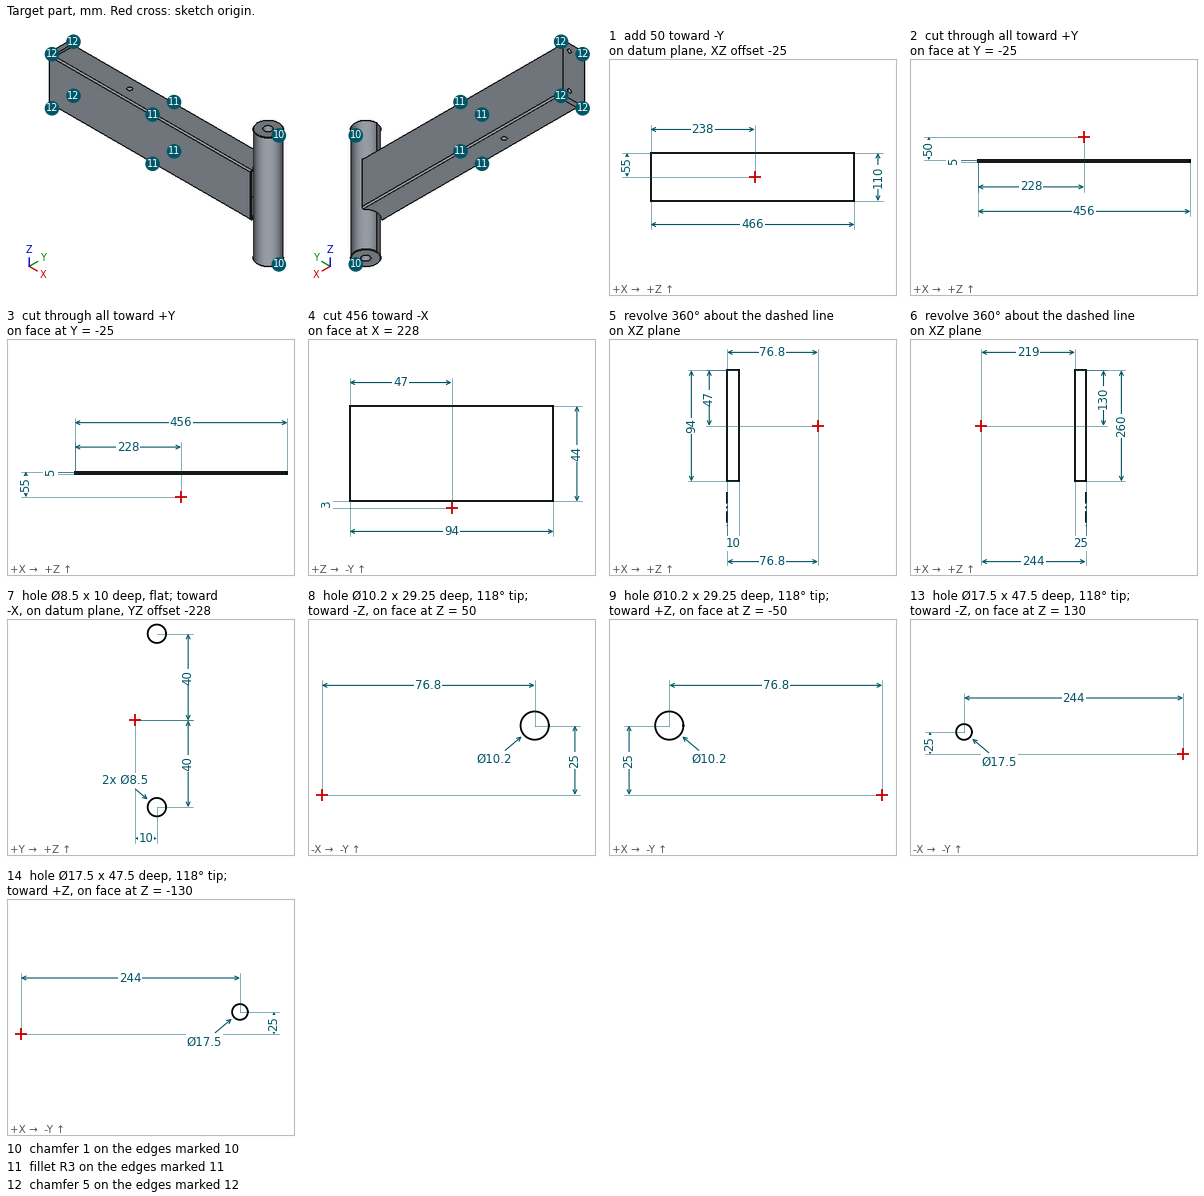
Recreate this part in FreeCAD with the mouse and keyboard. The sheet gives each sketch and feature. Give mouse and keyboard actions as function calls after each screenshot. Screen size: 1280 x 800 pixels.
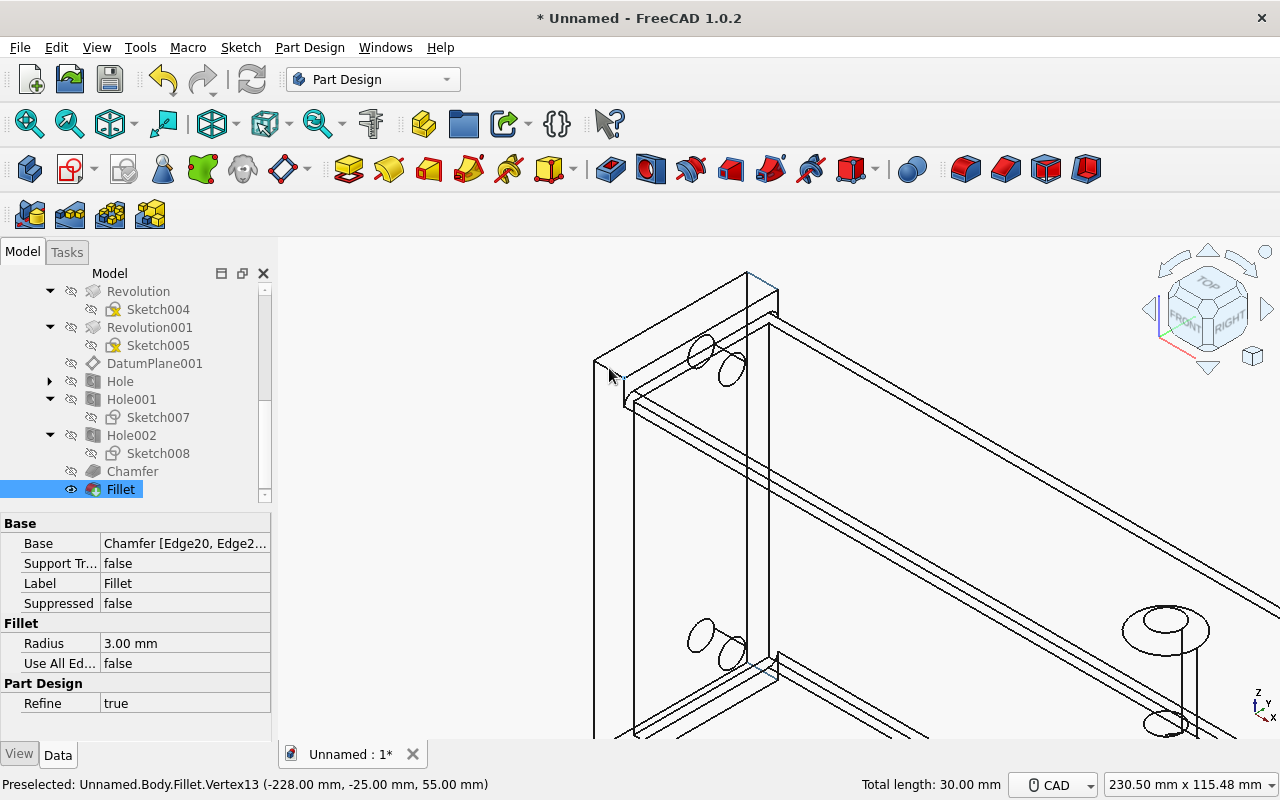
click(609, 368, ctrl)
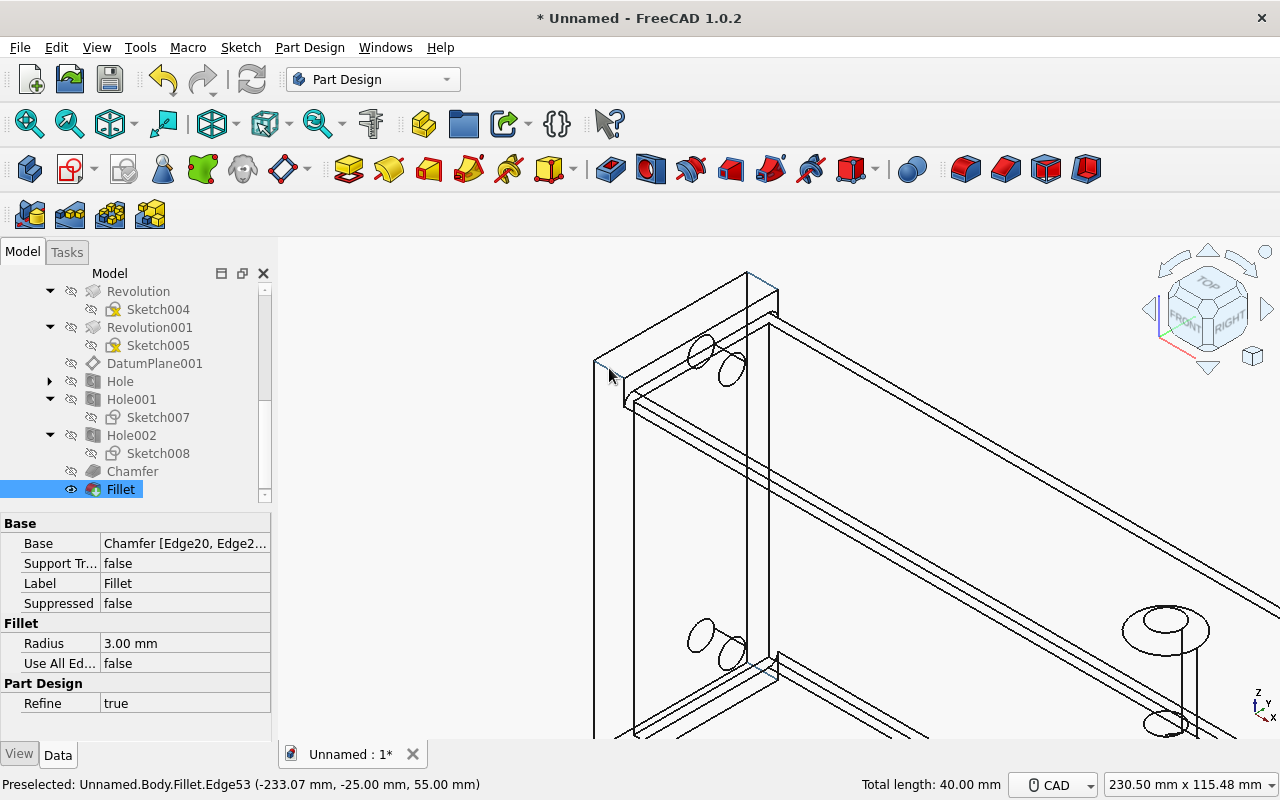
key(v)
key(1)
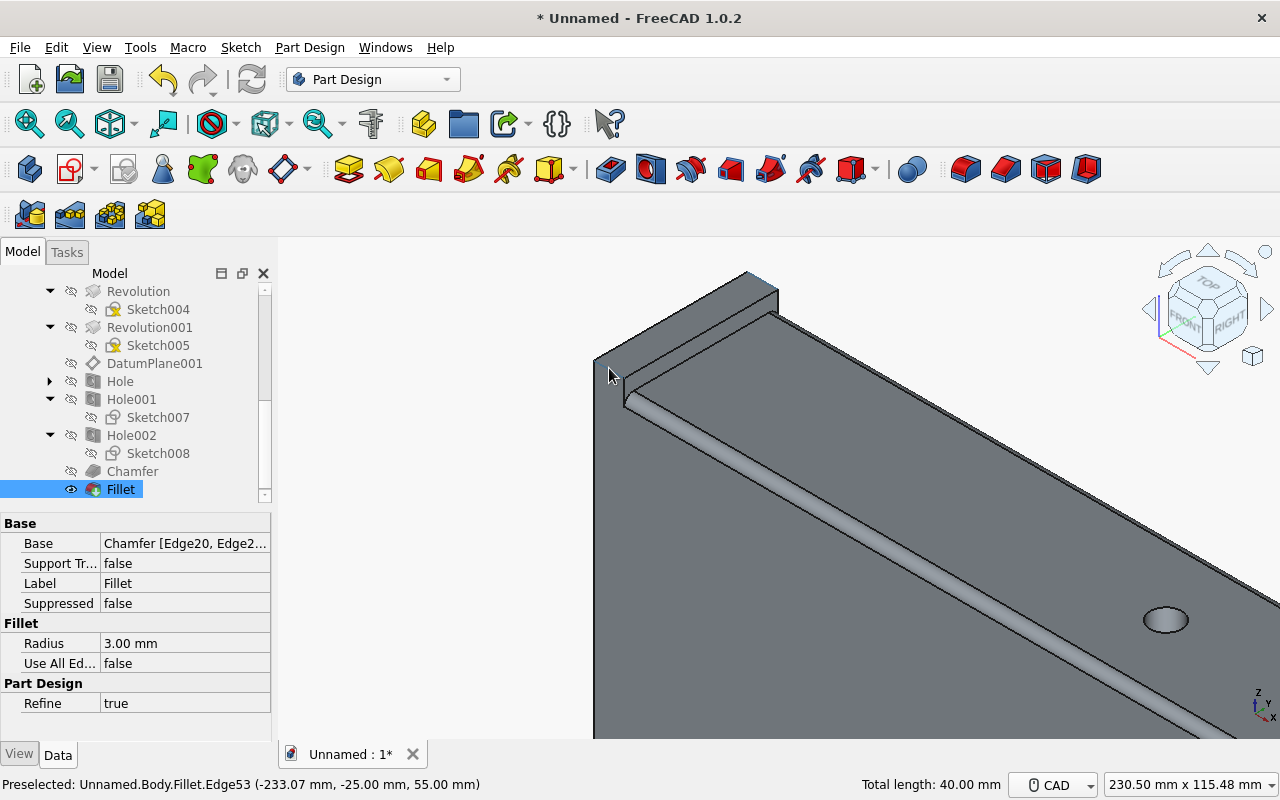
click(1006, 170)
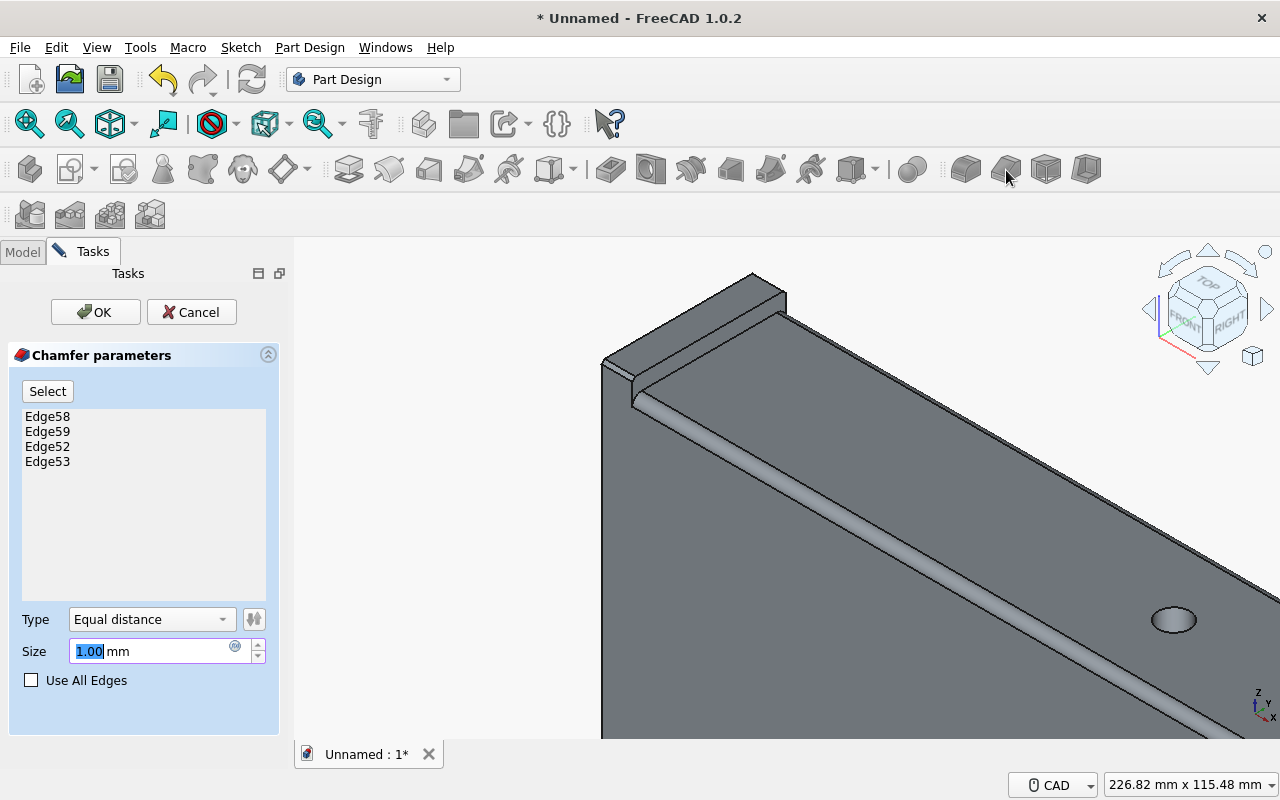
text(5)
key(Tab)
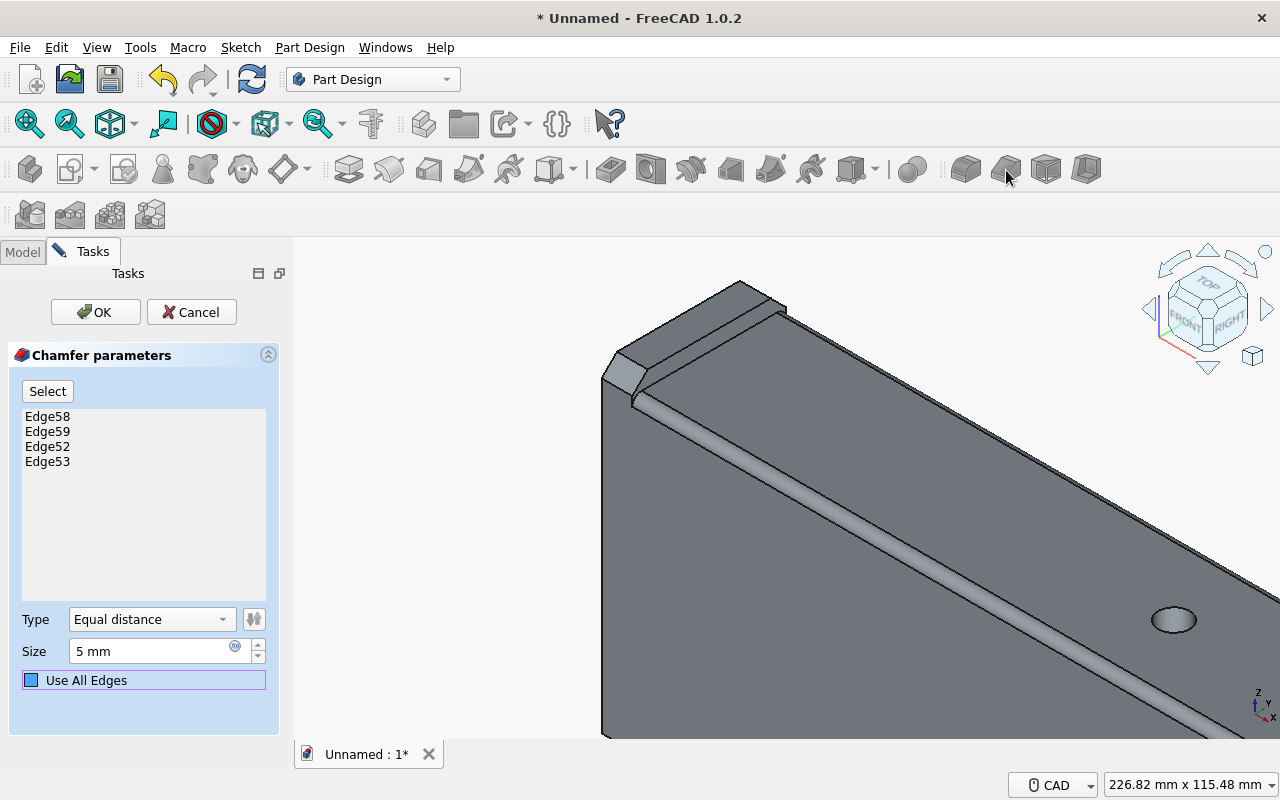
click(96, 312)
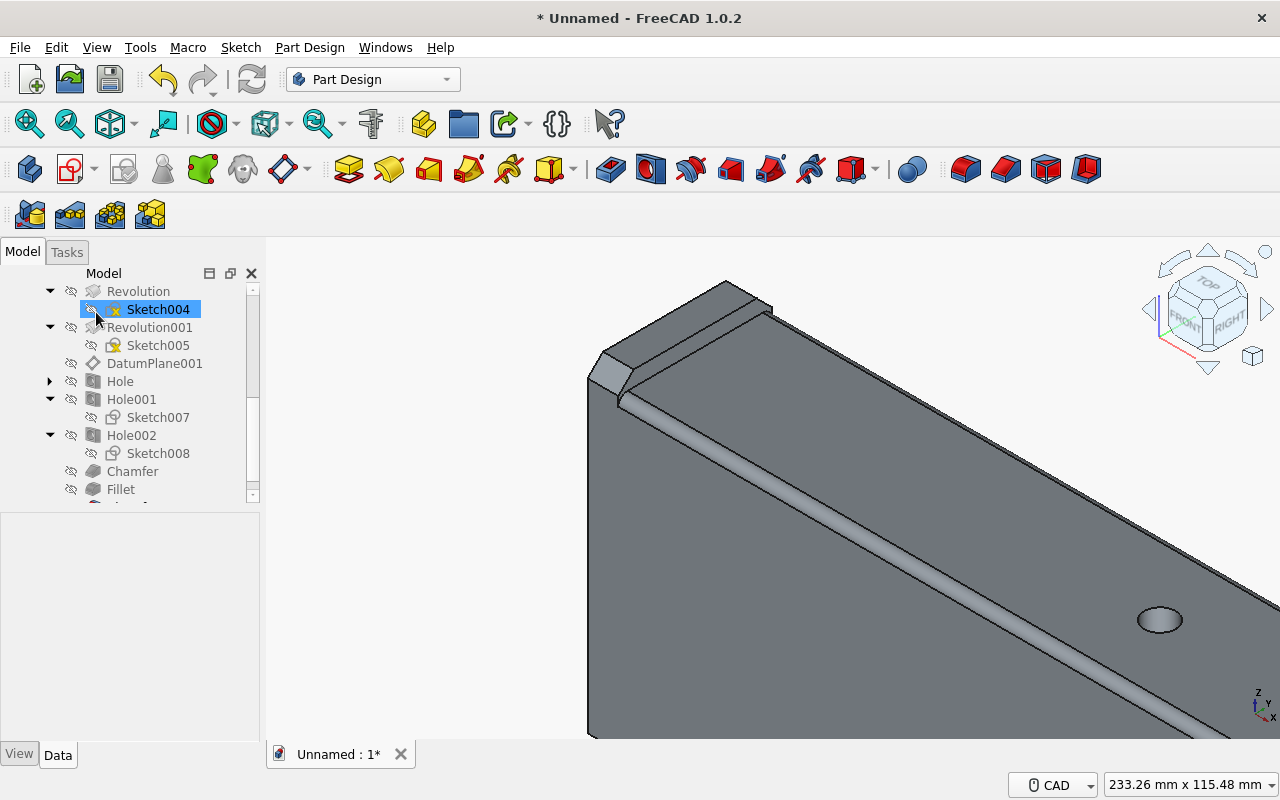
click(30, 124)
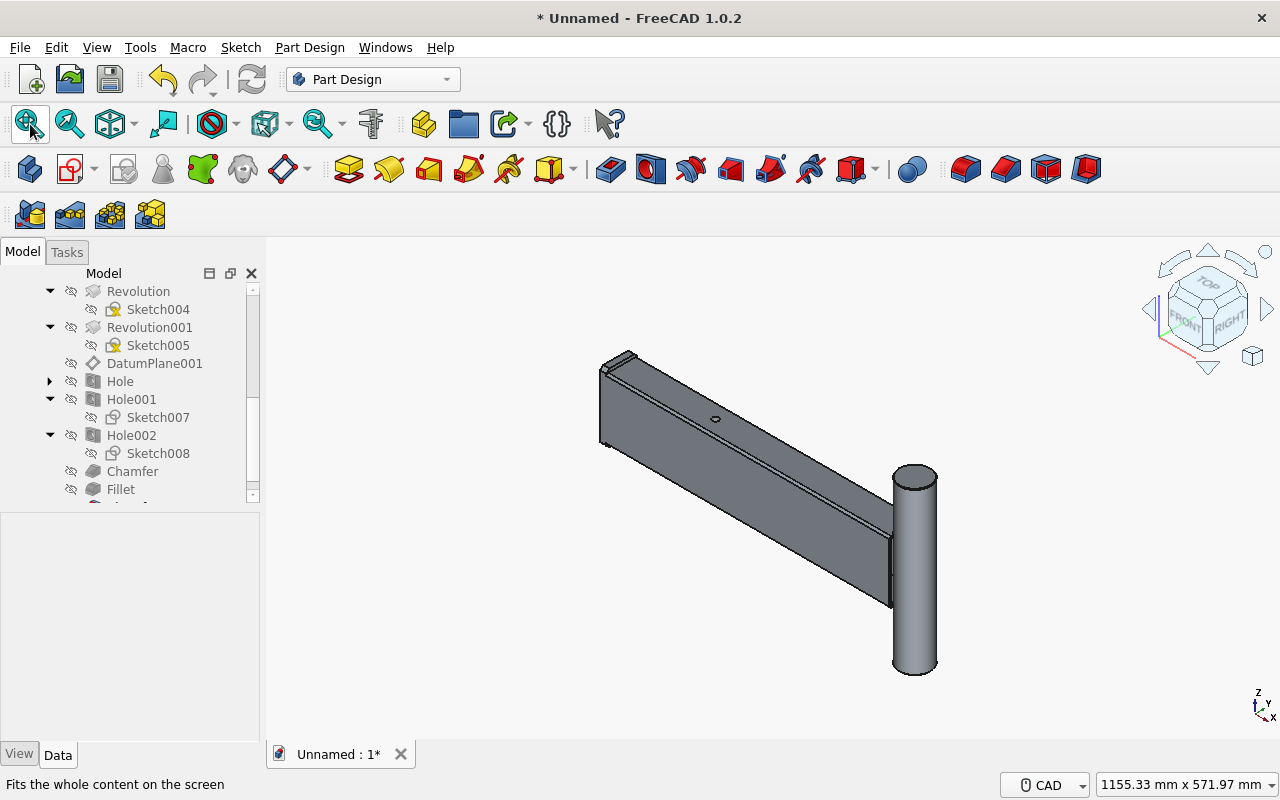
click(915, 476)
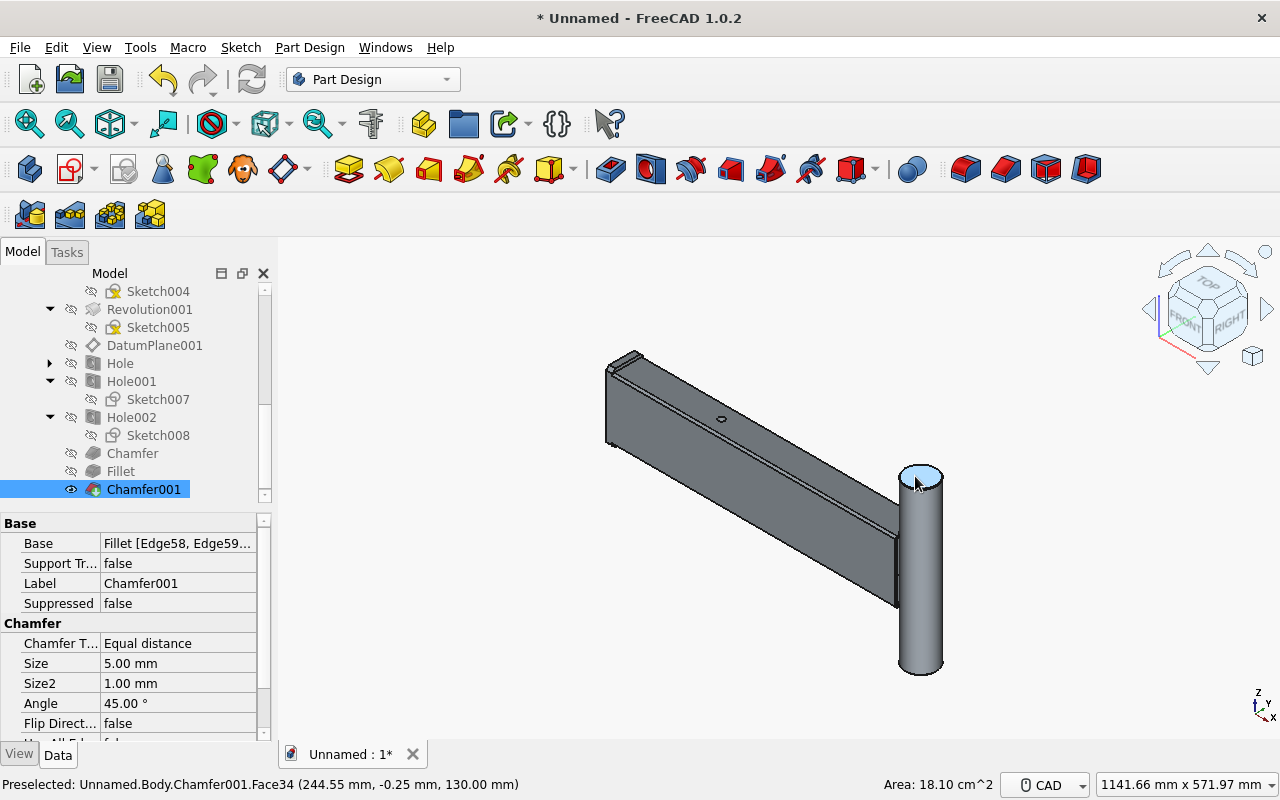
click(70, 170)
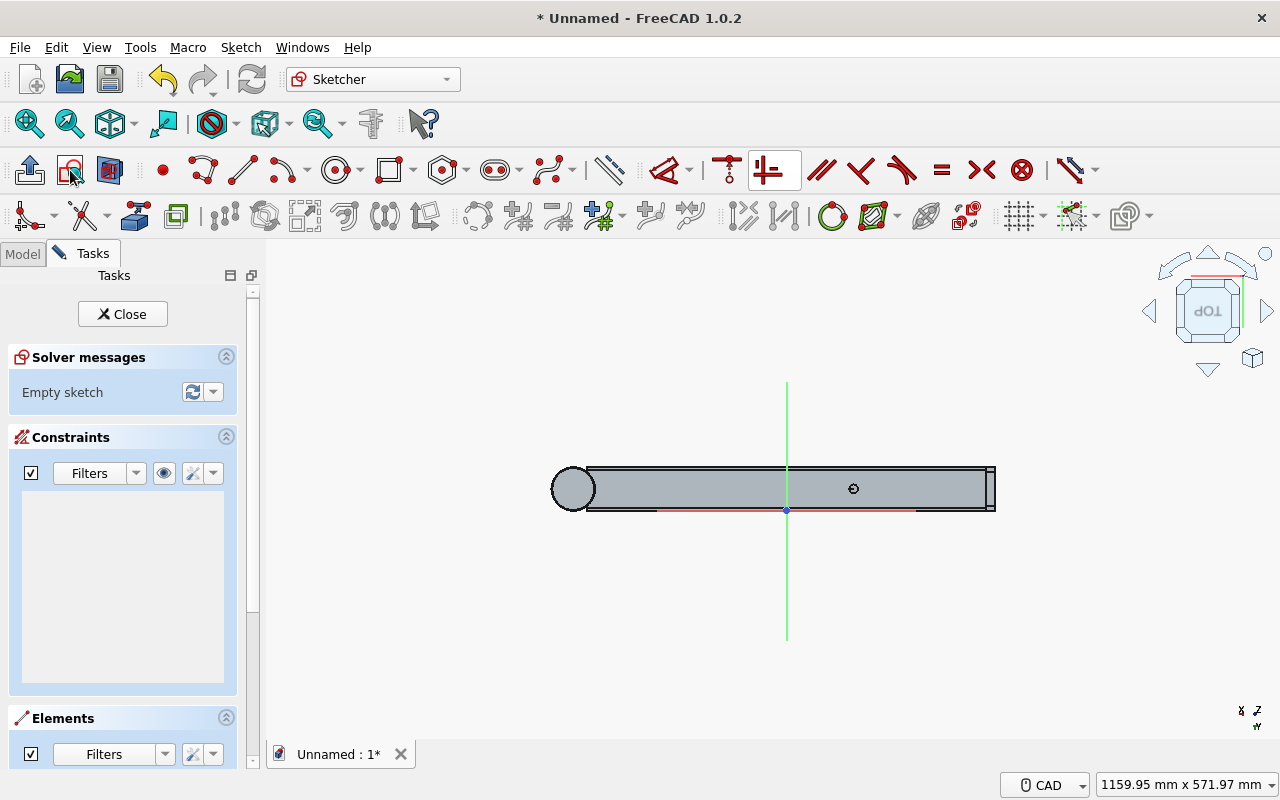
scroll(566, 489, up, 15)